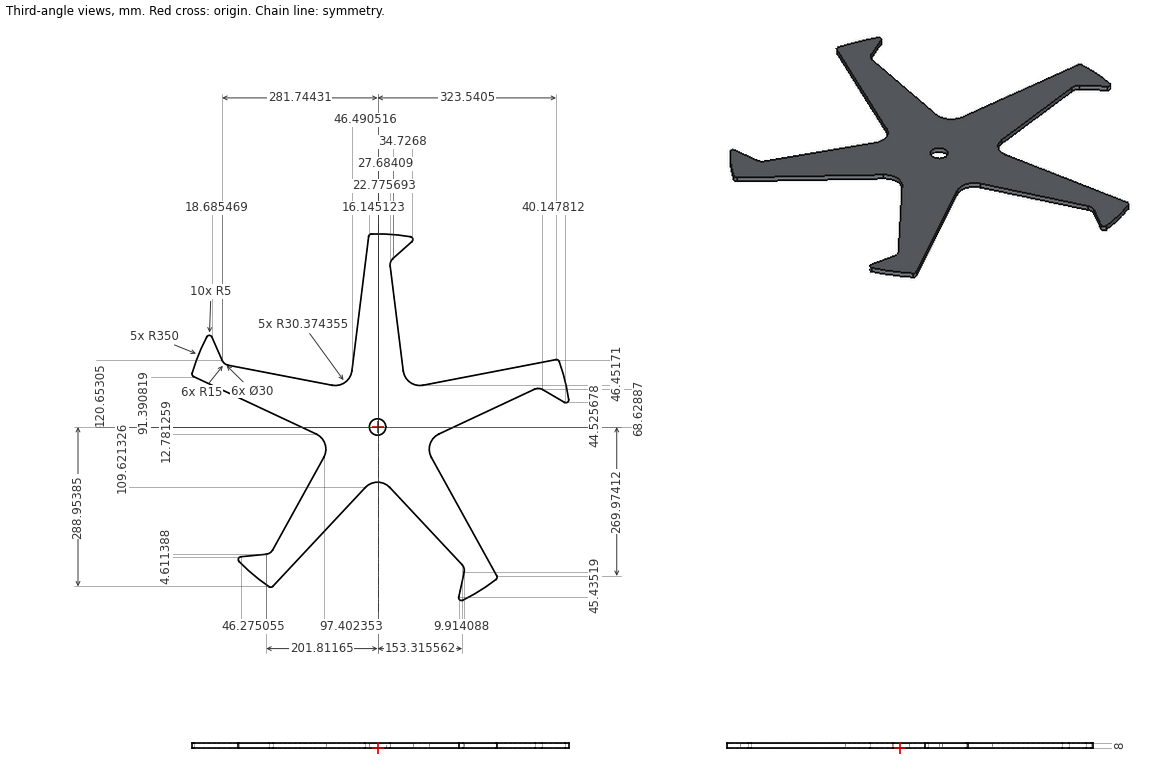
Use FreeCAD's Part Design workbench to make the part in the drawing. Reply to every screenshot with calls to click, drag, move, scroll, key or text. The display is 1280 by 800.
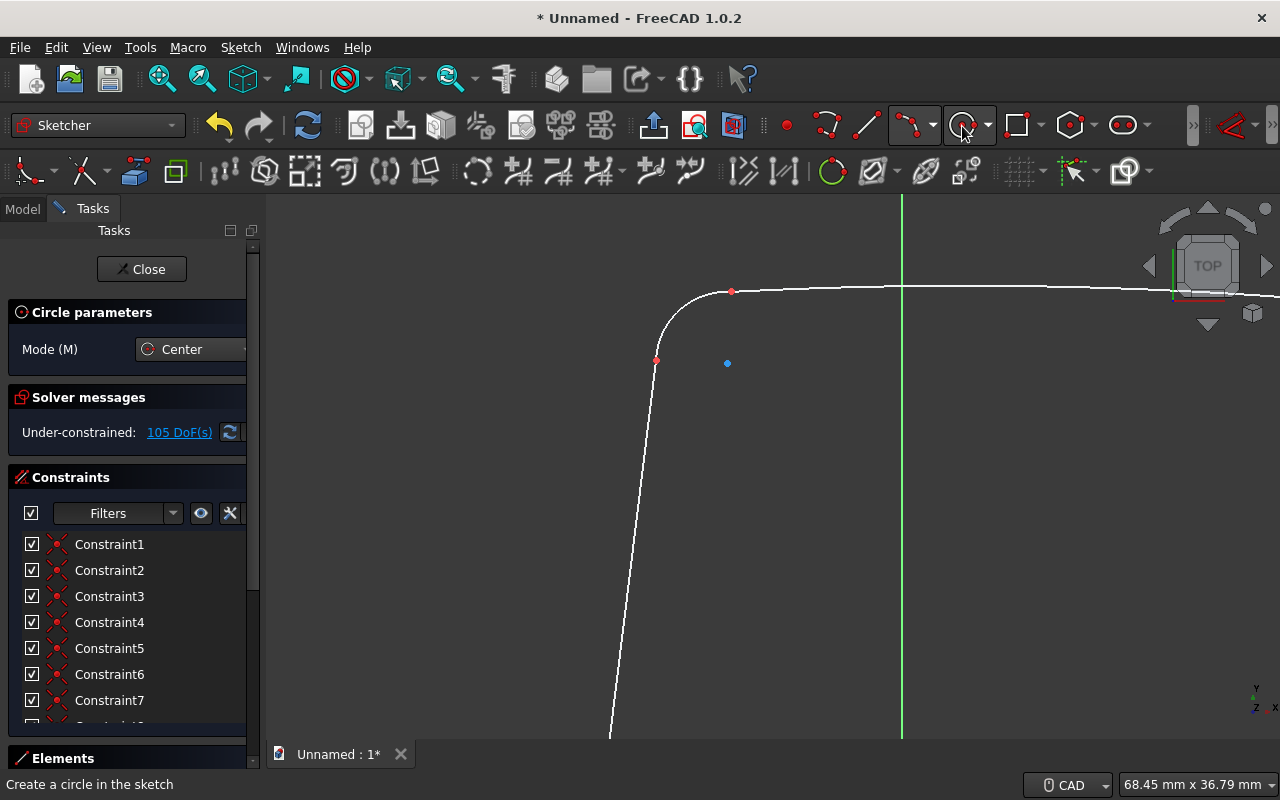
scroll(693, 265, down, 16)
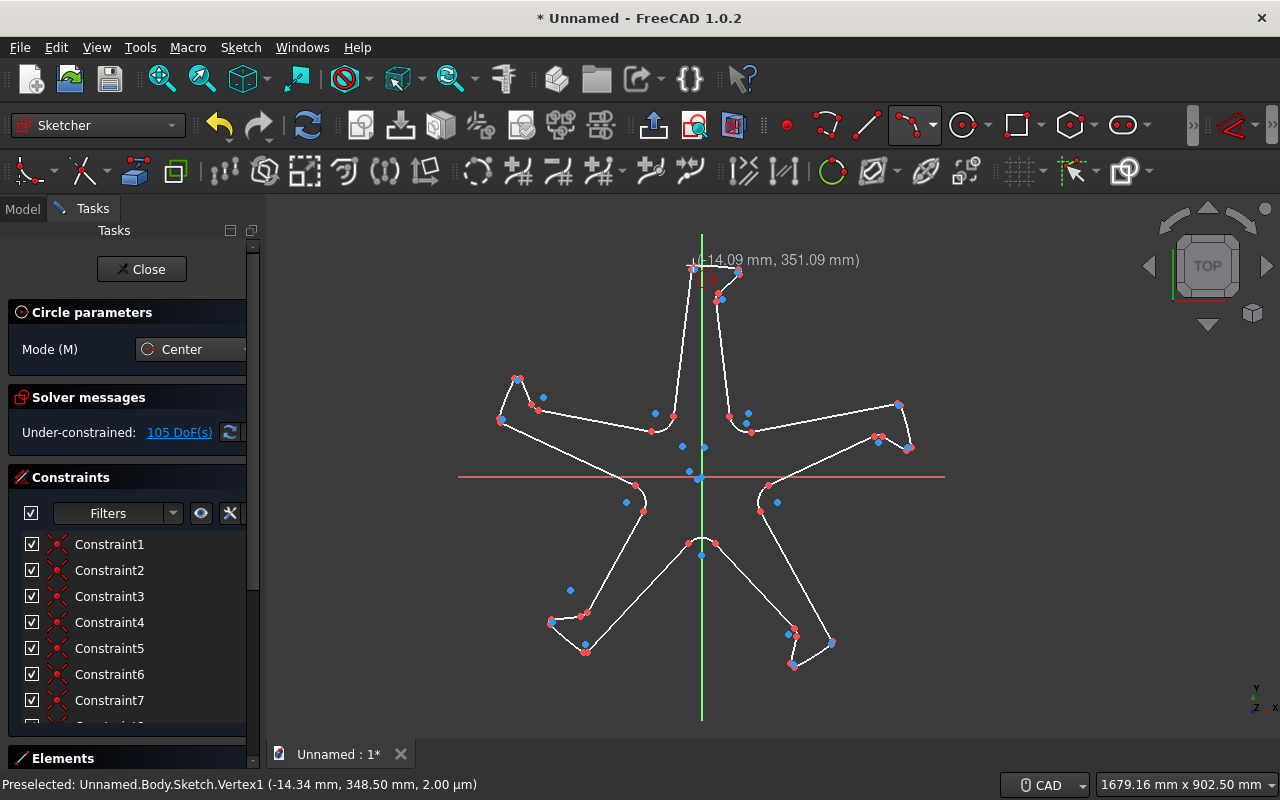
scroll(702, 477, up, 5)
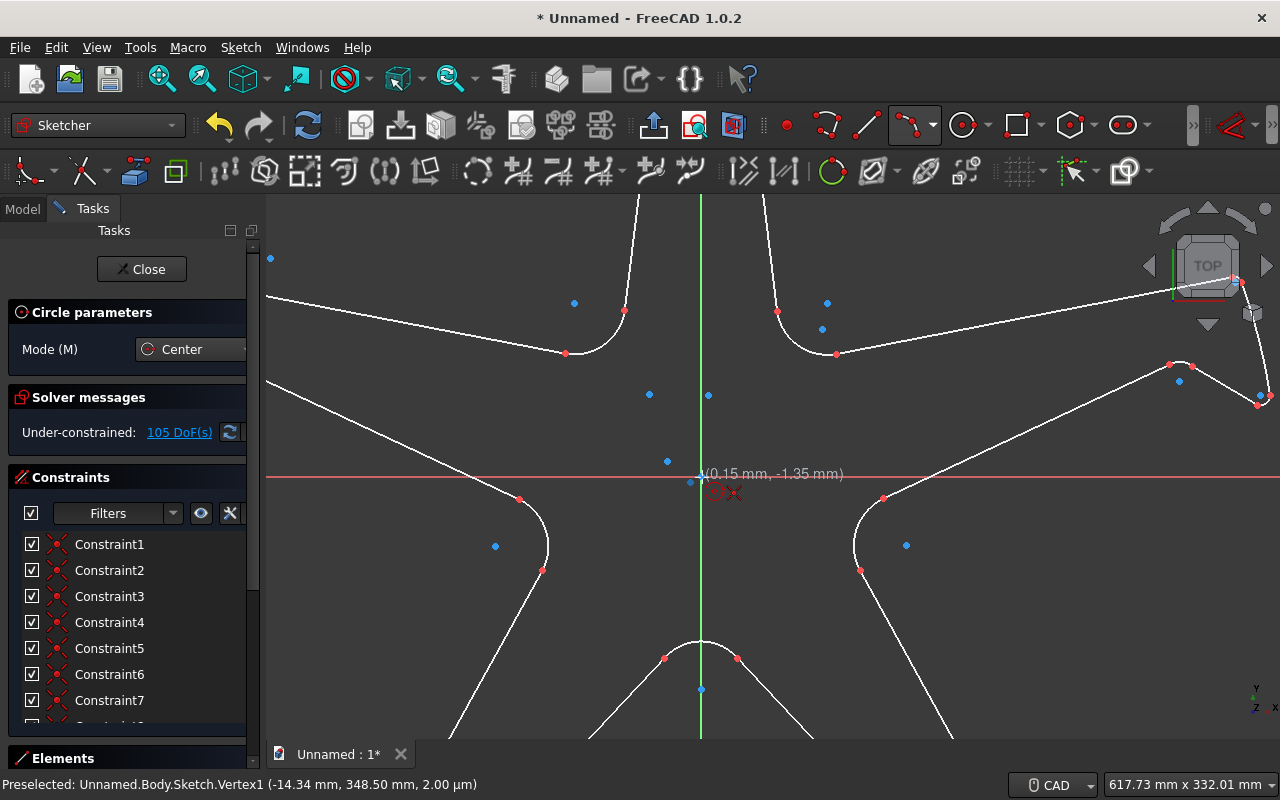
click(701, 477)
click(718, 459)
key(Escape)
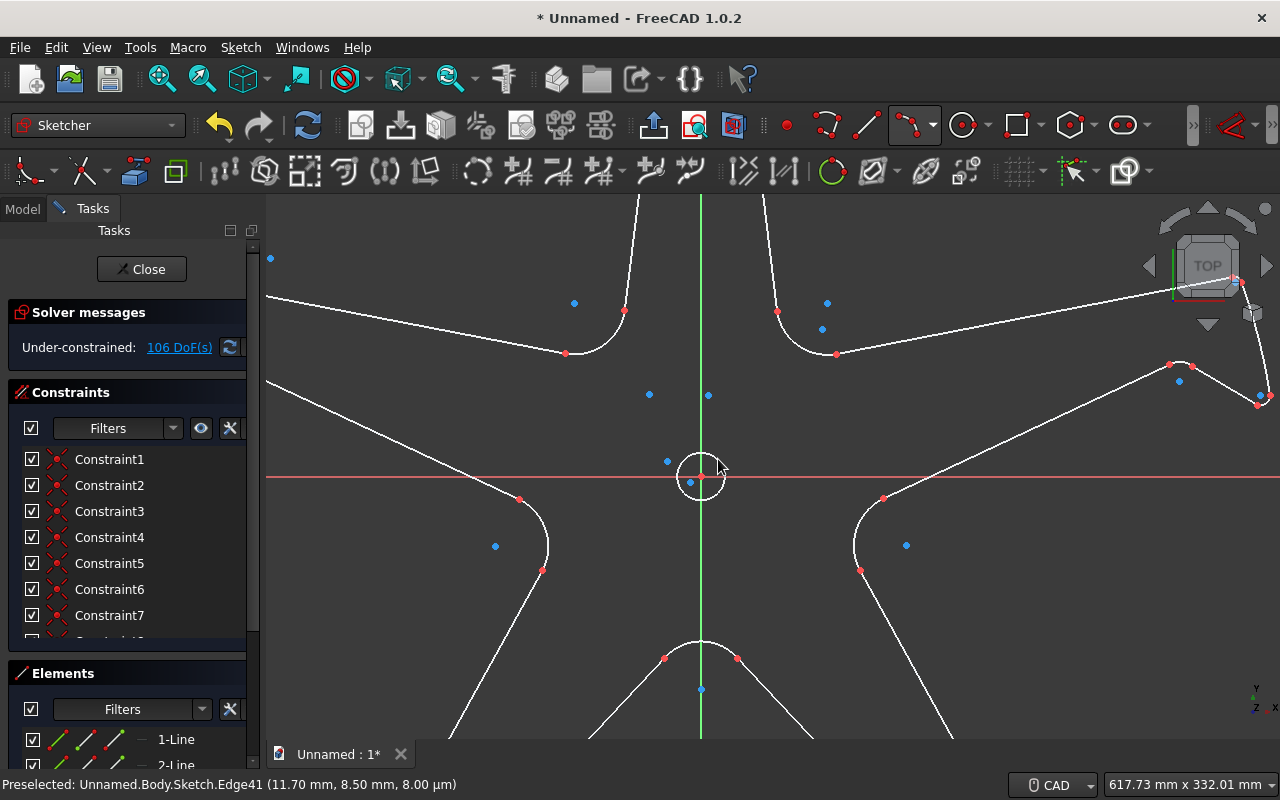
click(635, 231)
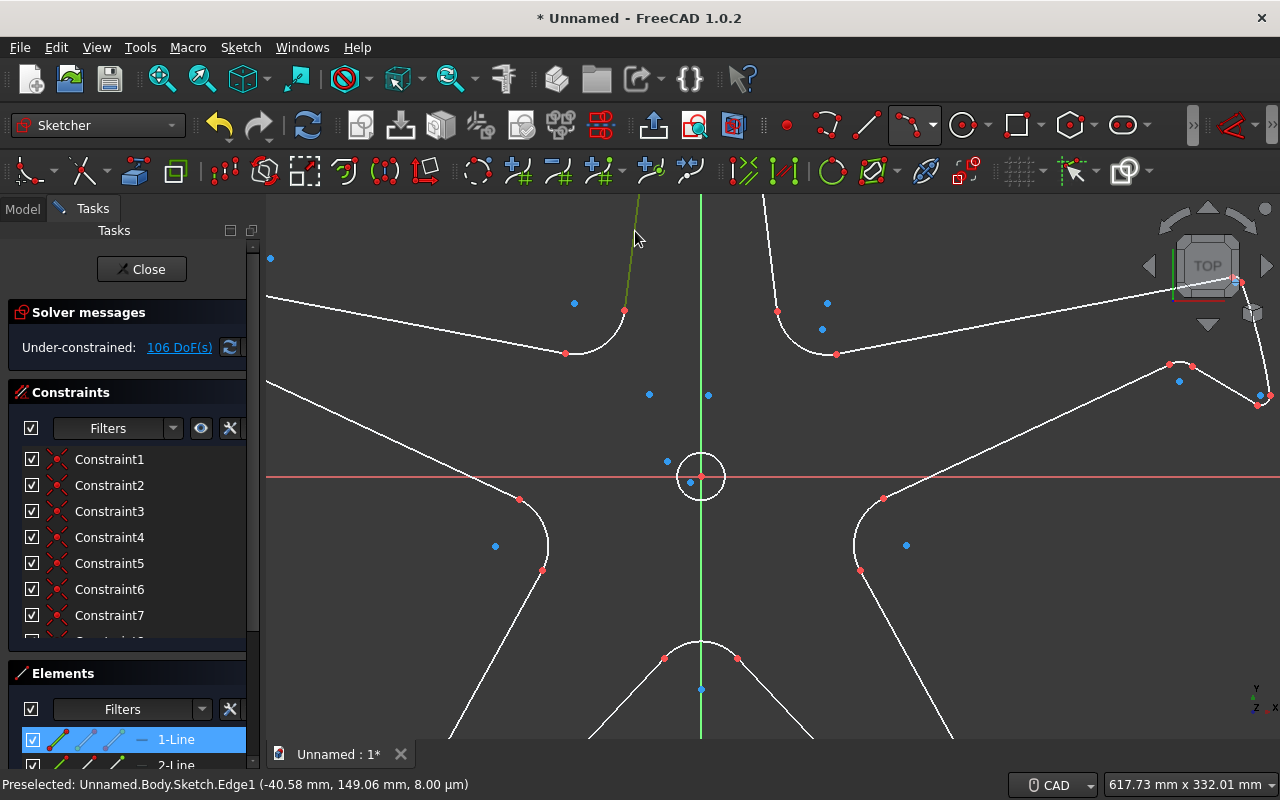
click(590, 352)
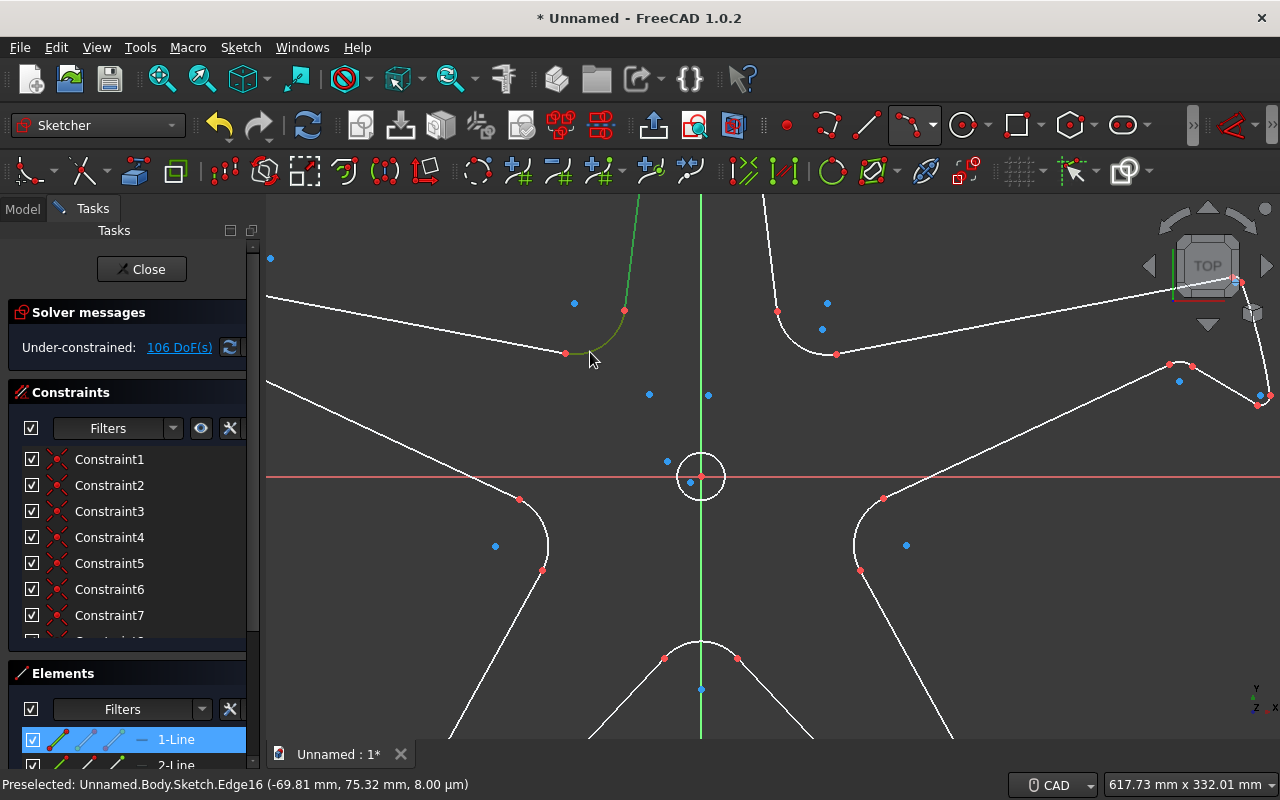
key(t)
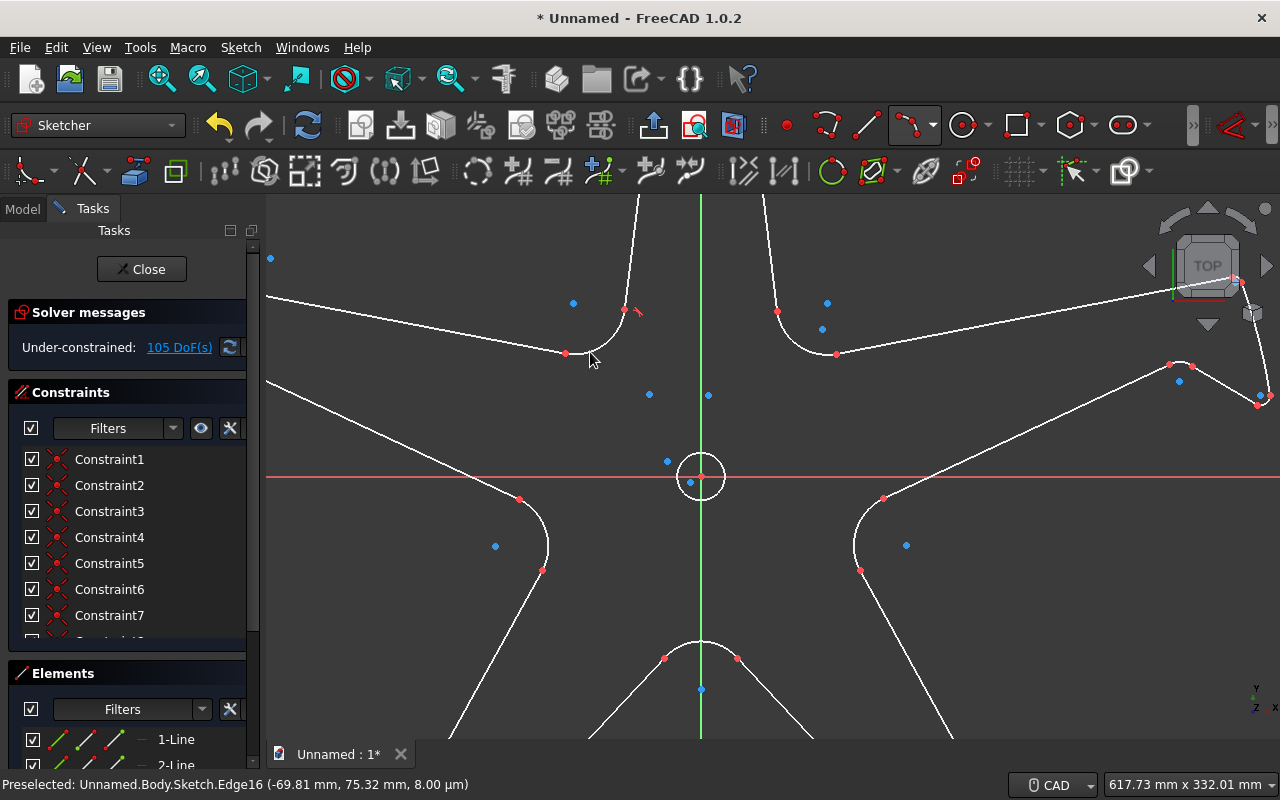
click(635, 230)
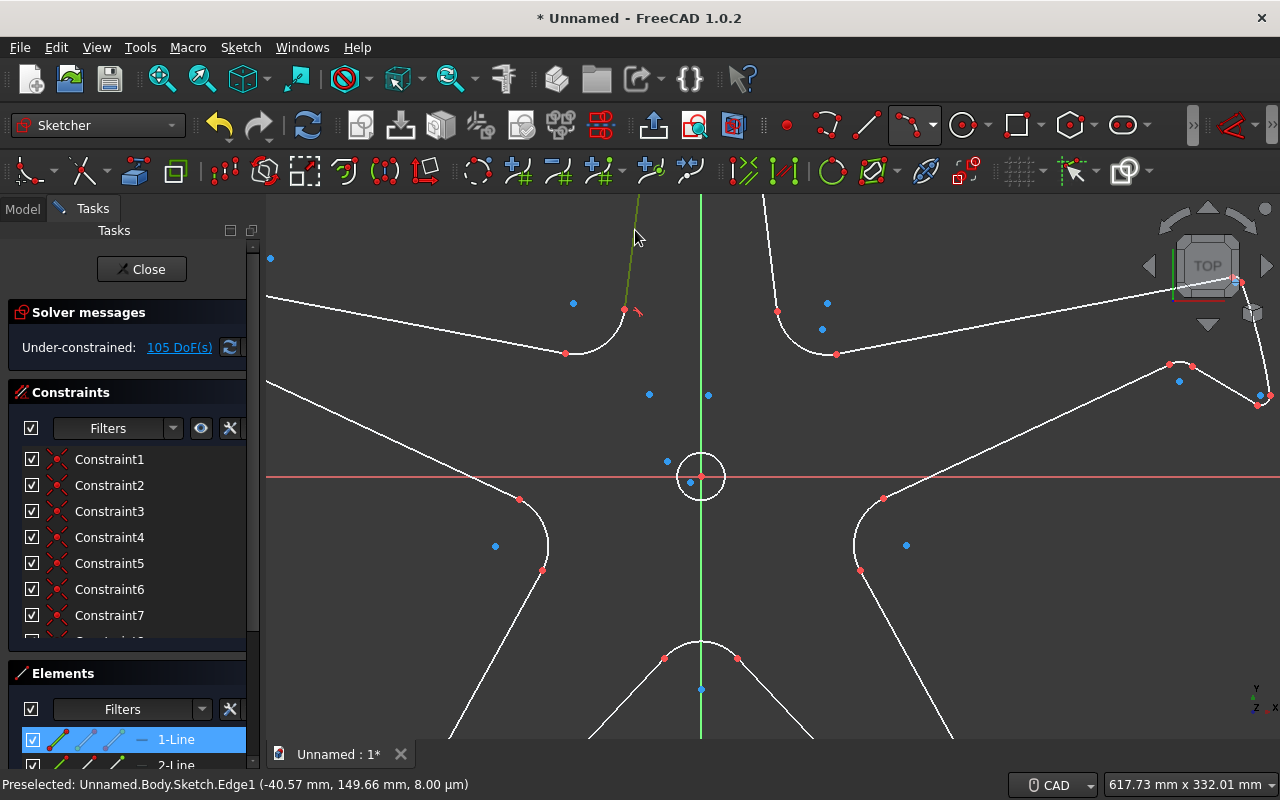
scroll(702, 475, down, 6)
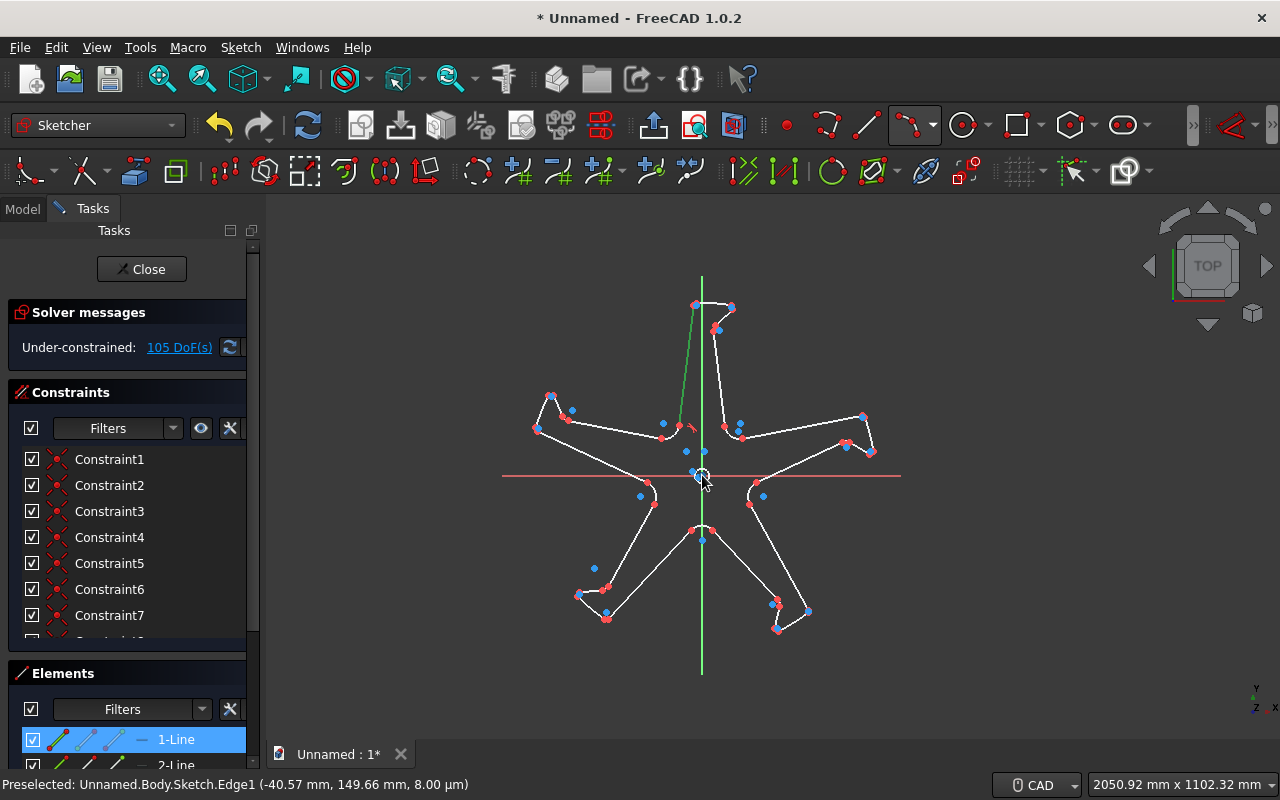
scroll(695, 304, up, 11)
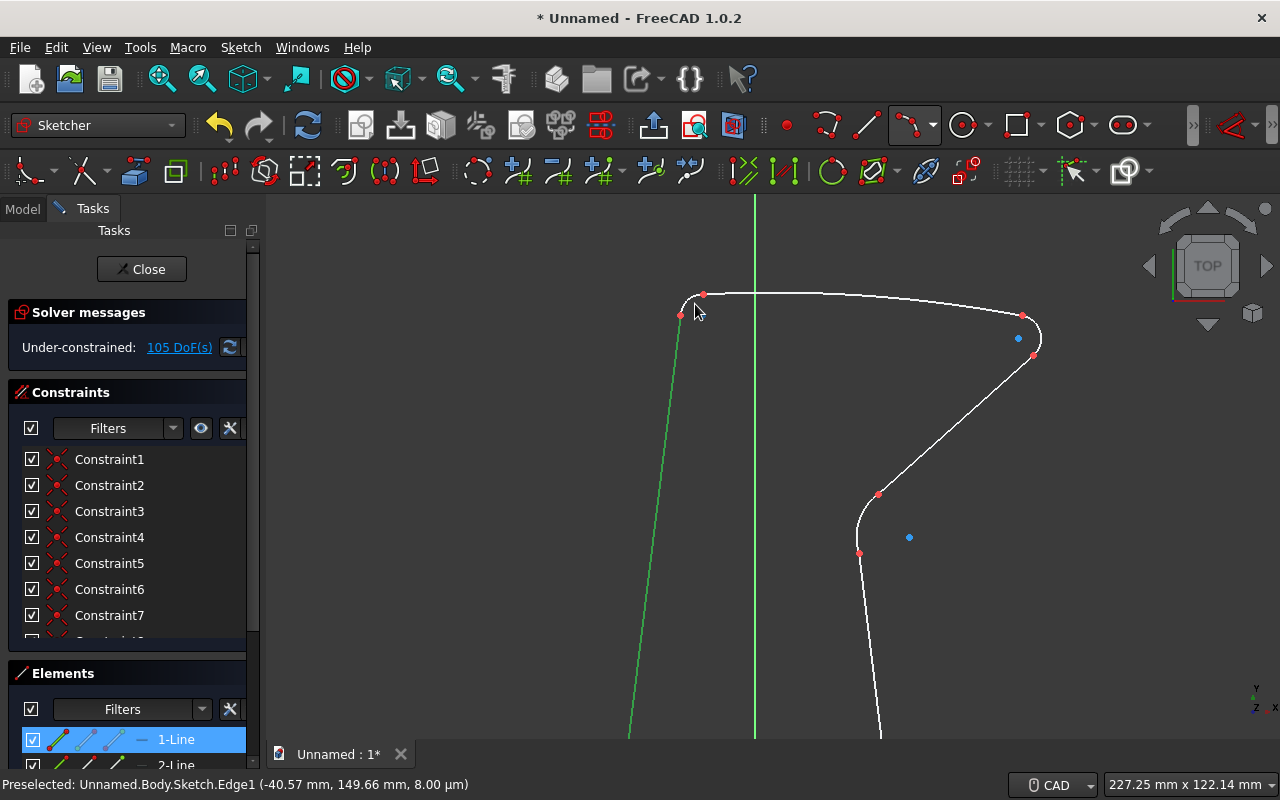
click(688, 300)